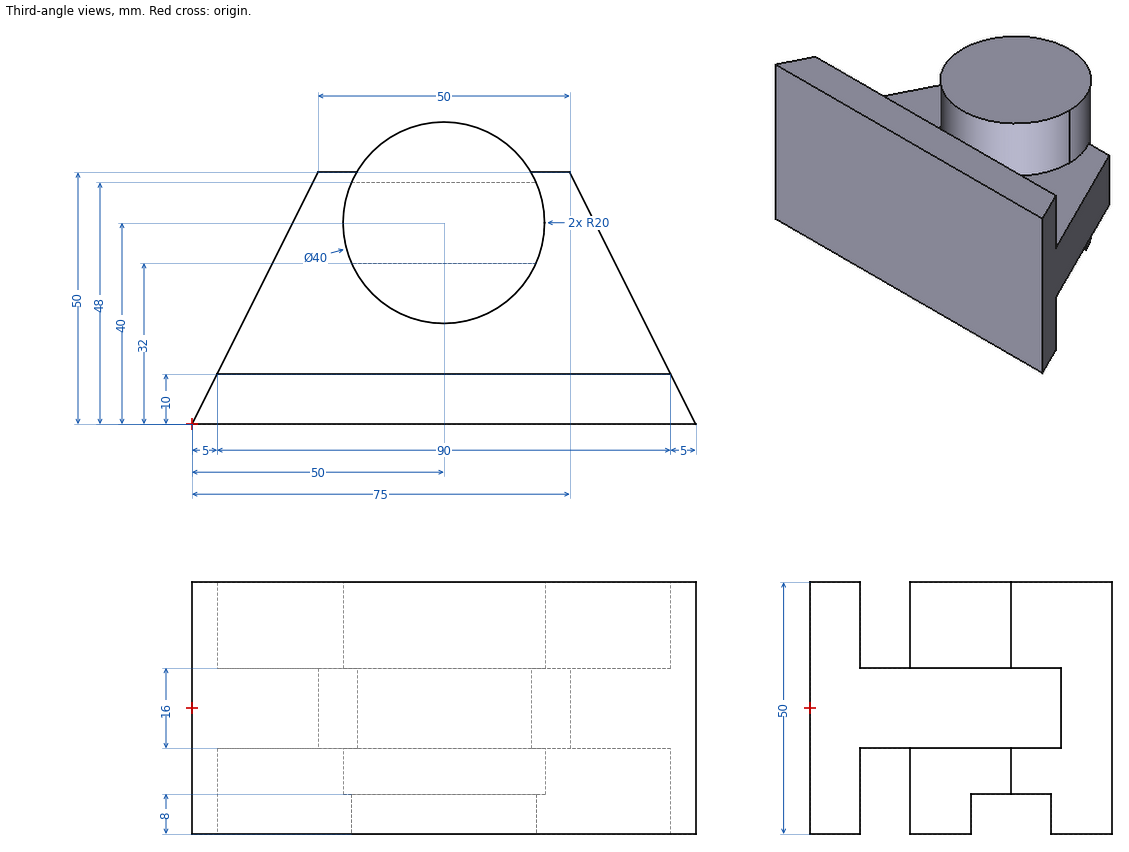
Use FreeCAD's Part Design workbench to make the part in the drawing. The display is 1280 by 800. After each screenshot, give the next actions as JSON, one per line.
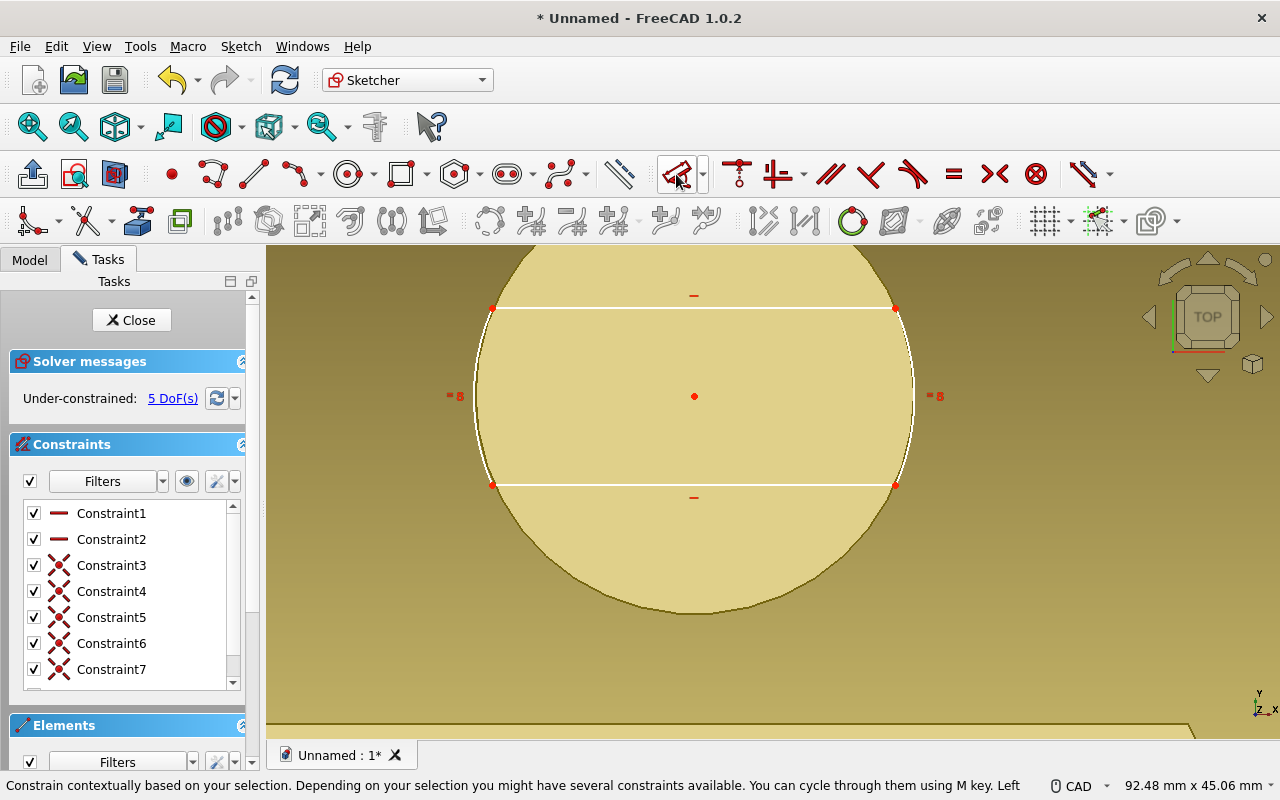
{"action": "left_click", "coordinate": [911, 433]}
{"action": "left_click", "coordinate": [943, 438]}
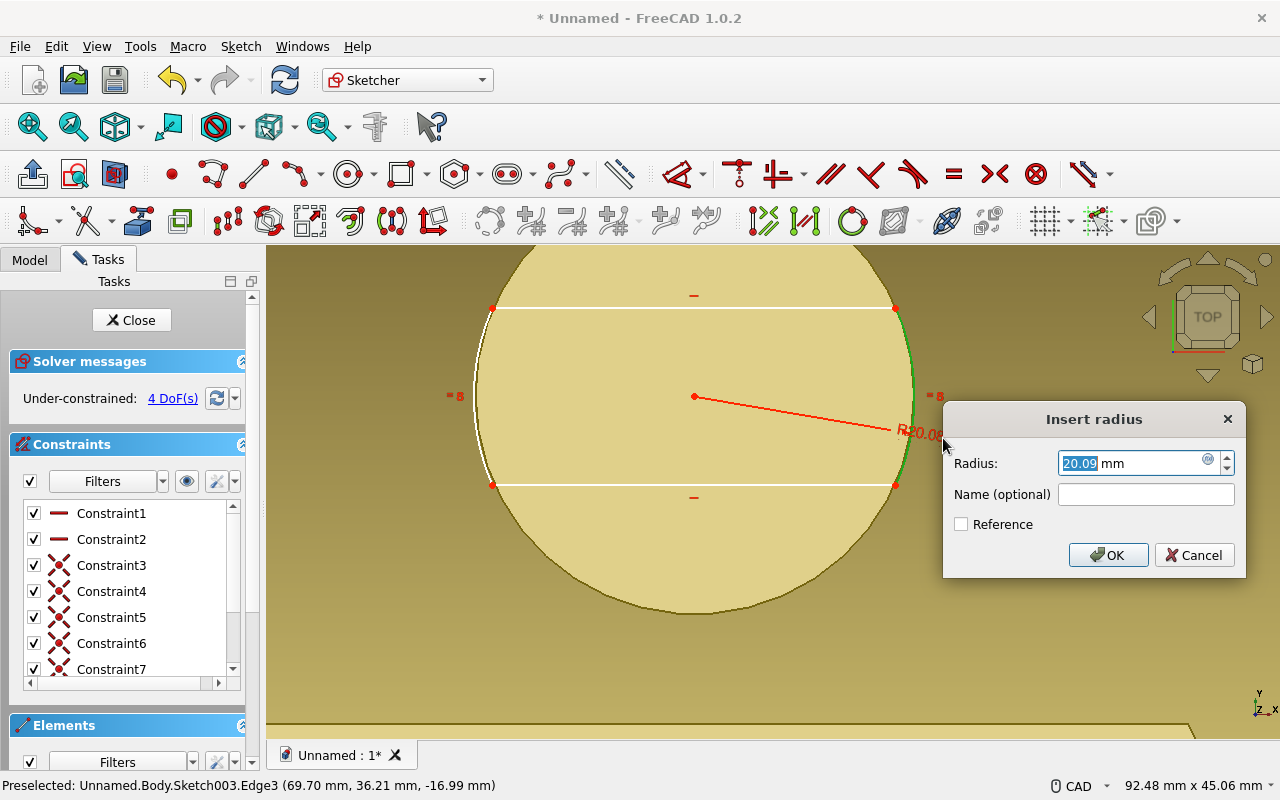
{"action": "type", "text": "20"}
{"action": "key", "text": "Return"}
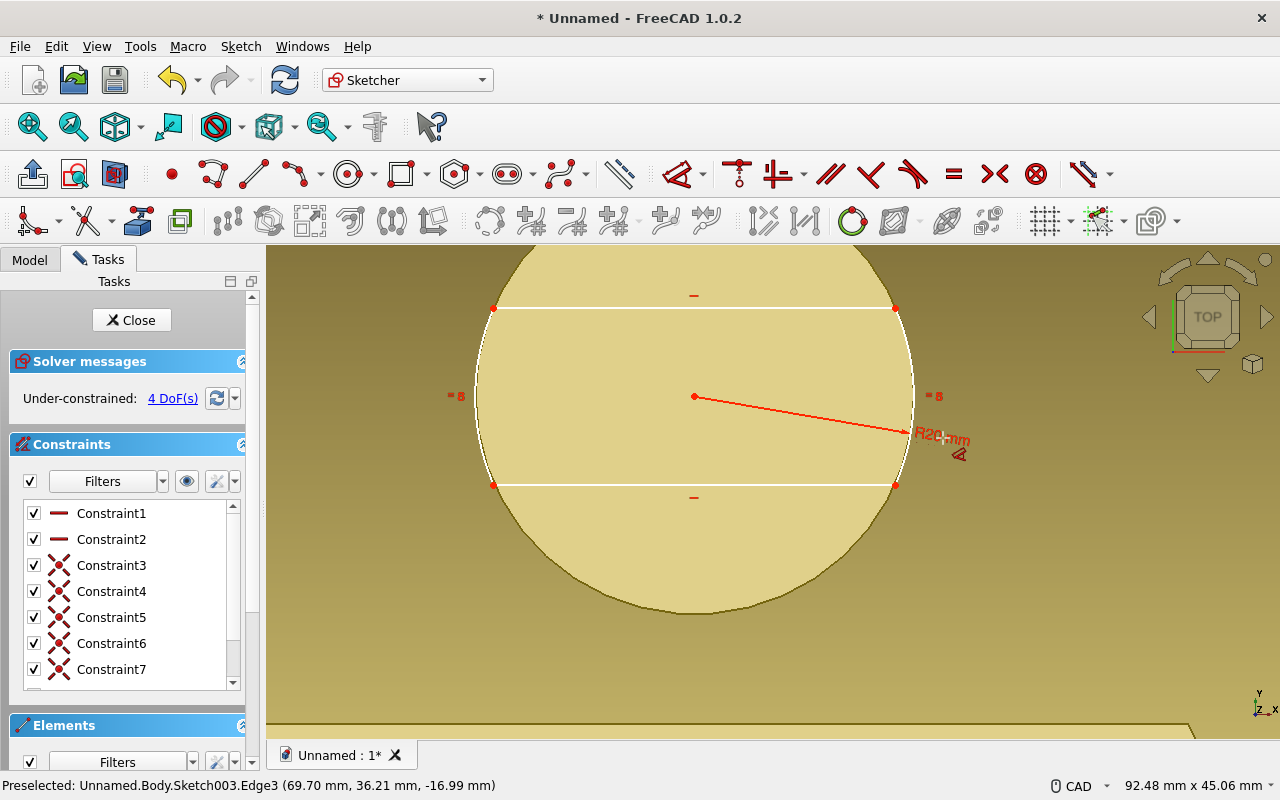
{"action": "left_click", "coordinate": [494, 308]}
{"action": "left_click", "coordinate": [528, 510]}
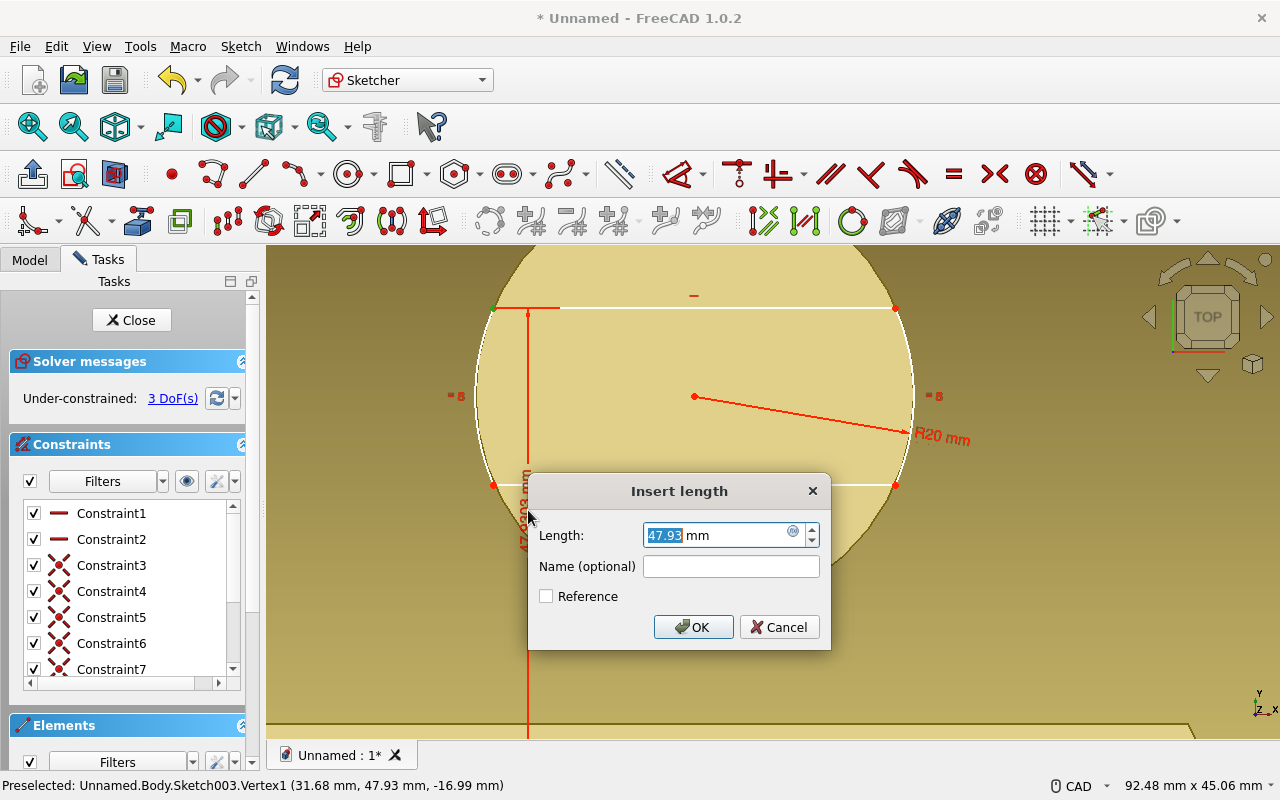
{"action": "type", "text": "48"}
{"action": "key", "text": "Return"}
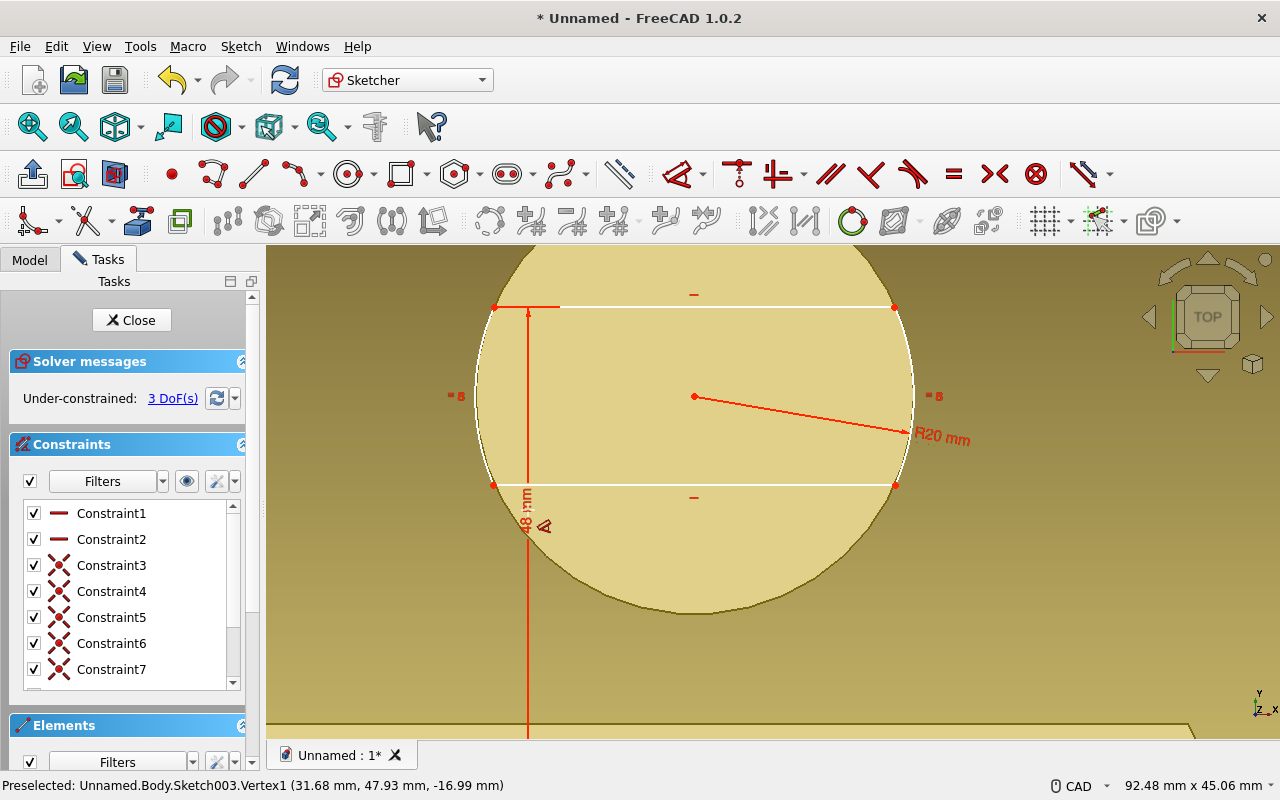
{"action": "left_click", "coordinate": [895, 485]}
{"action": "left_click", "coordinate": [929, 598]}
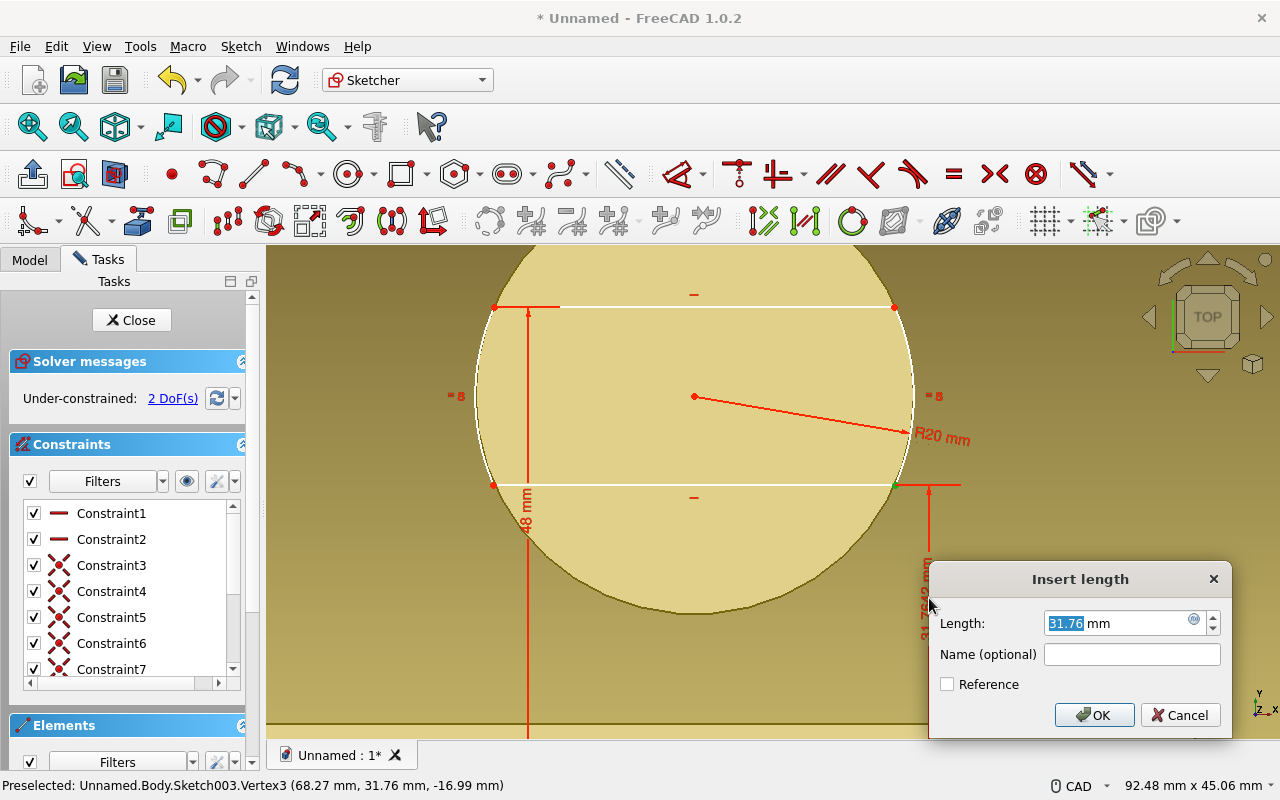
{"action": "type", "text": "32"}
{"action": "key", "text": "Return"}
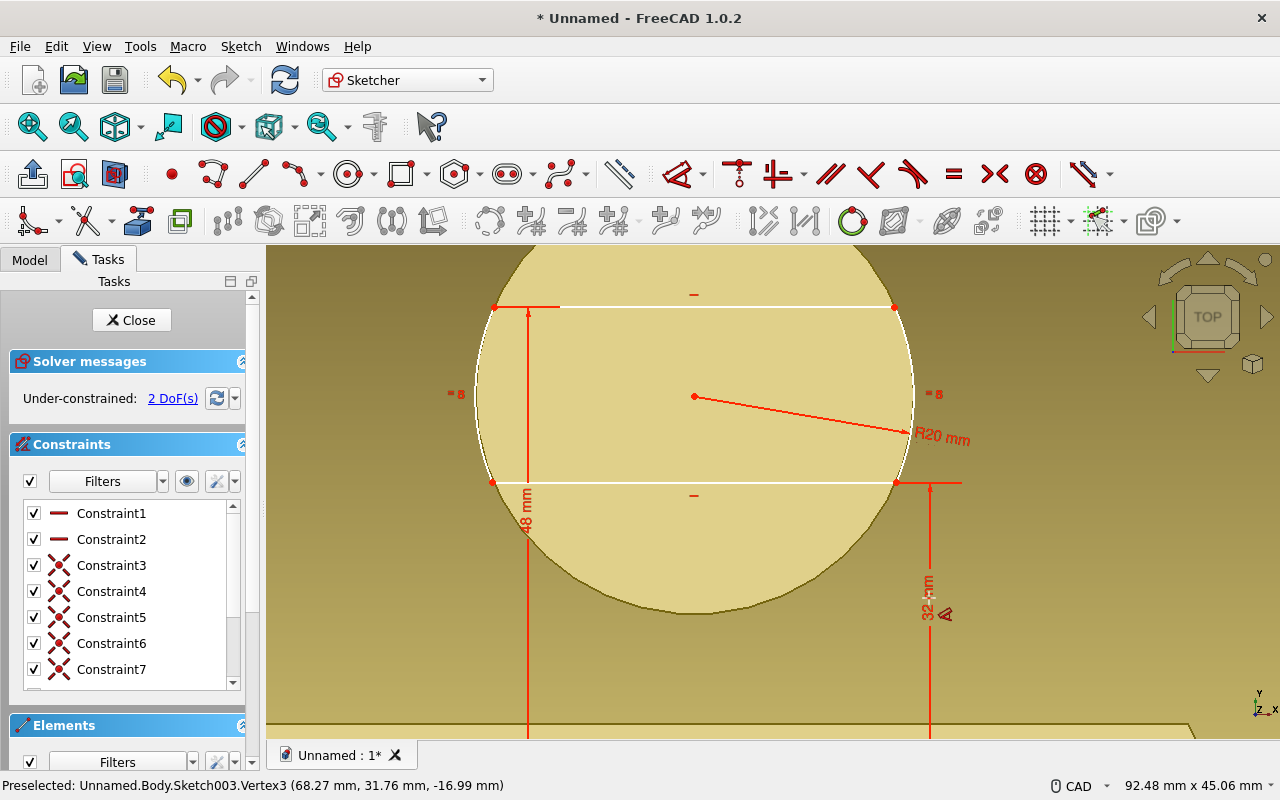
{"action": "left_click", "coordinate": [695, 397]}
{"action": "left_click", "coordinate": [494, 363]}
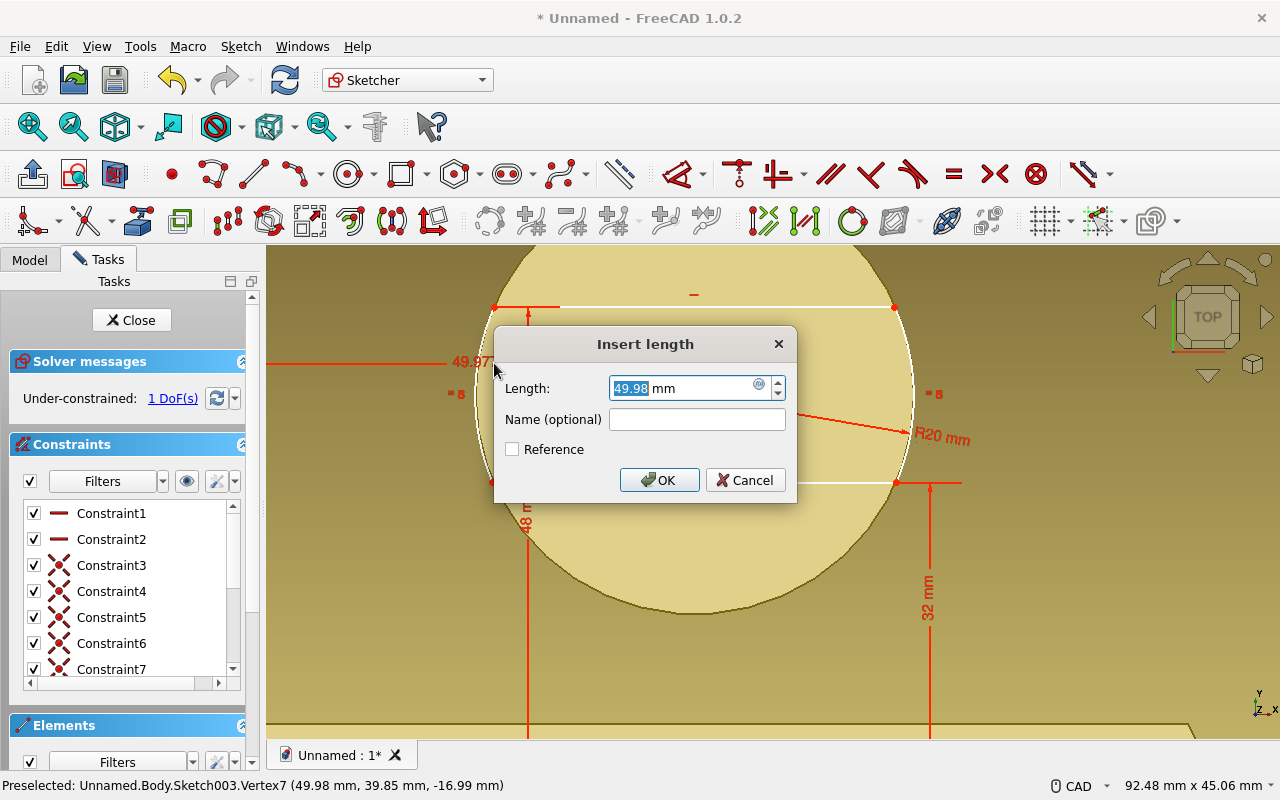
{"action": "type", "text": "50"}
{"action": "key", "text": "Return"}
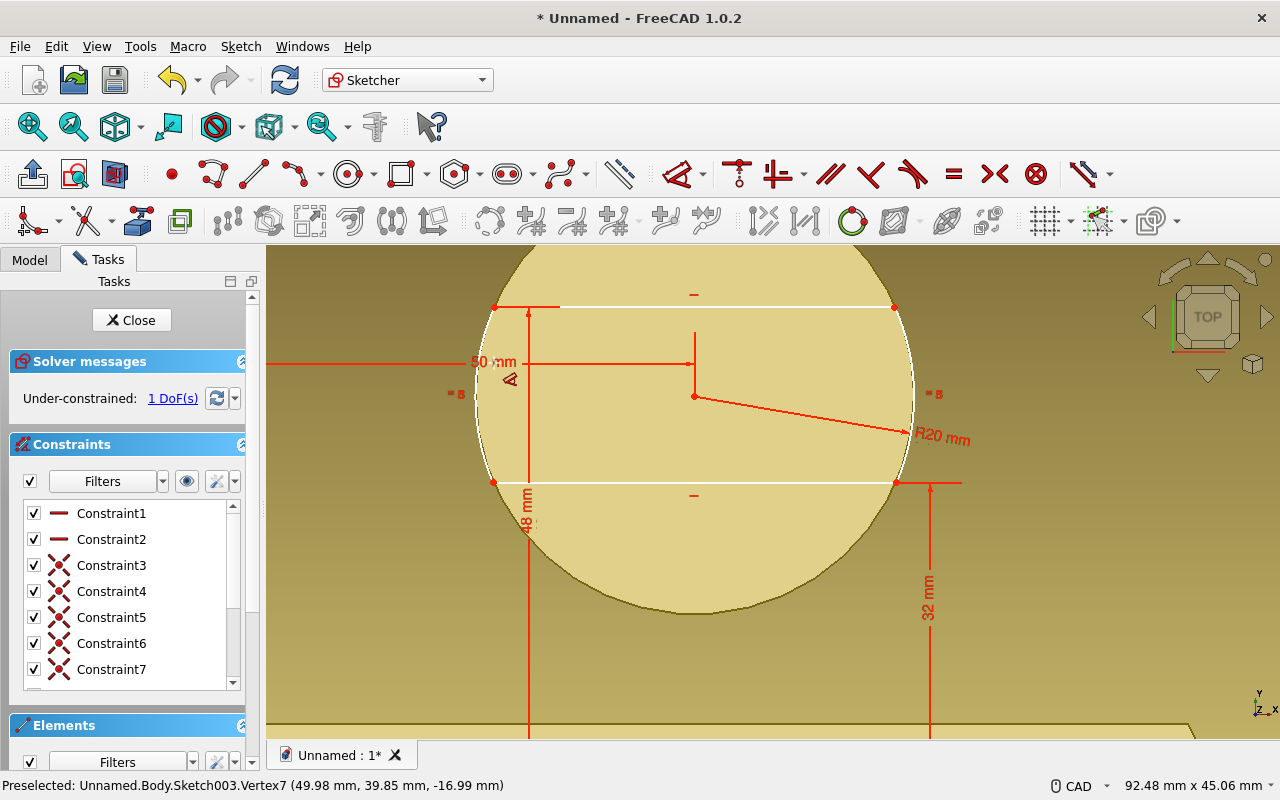
{"action": "left_click", "coordinate": [695, 397]}
{"action": "left_click", "coordinate": [729, 554]}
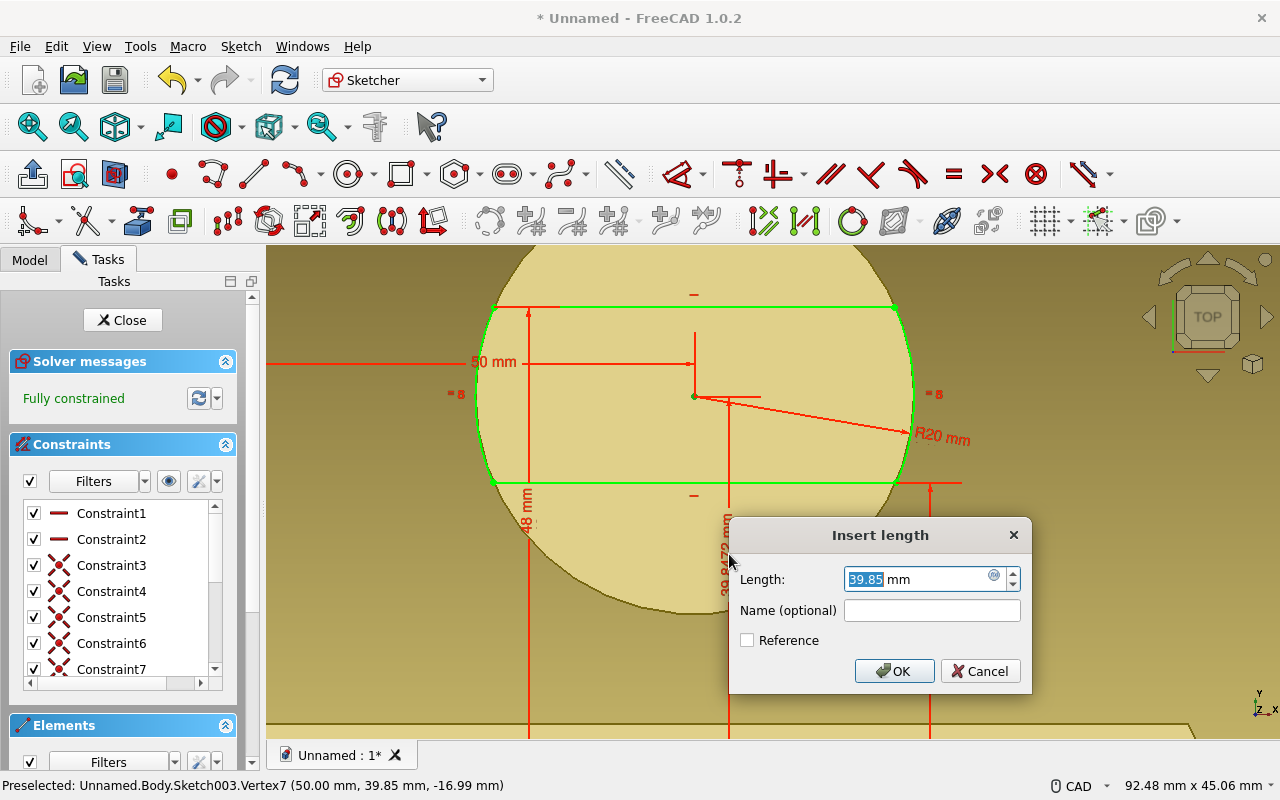
{"action": "type", "text": "40"}
{"action": "key", "text": "Return"}
{"action": "key", "text": "Escape"}